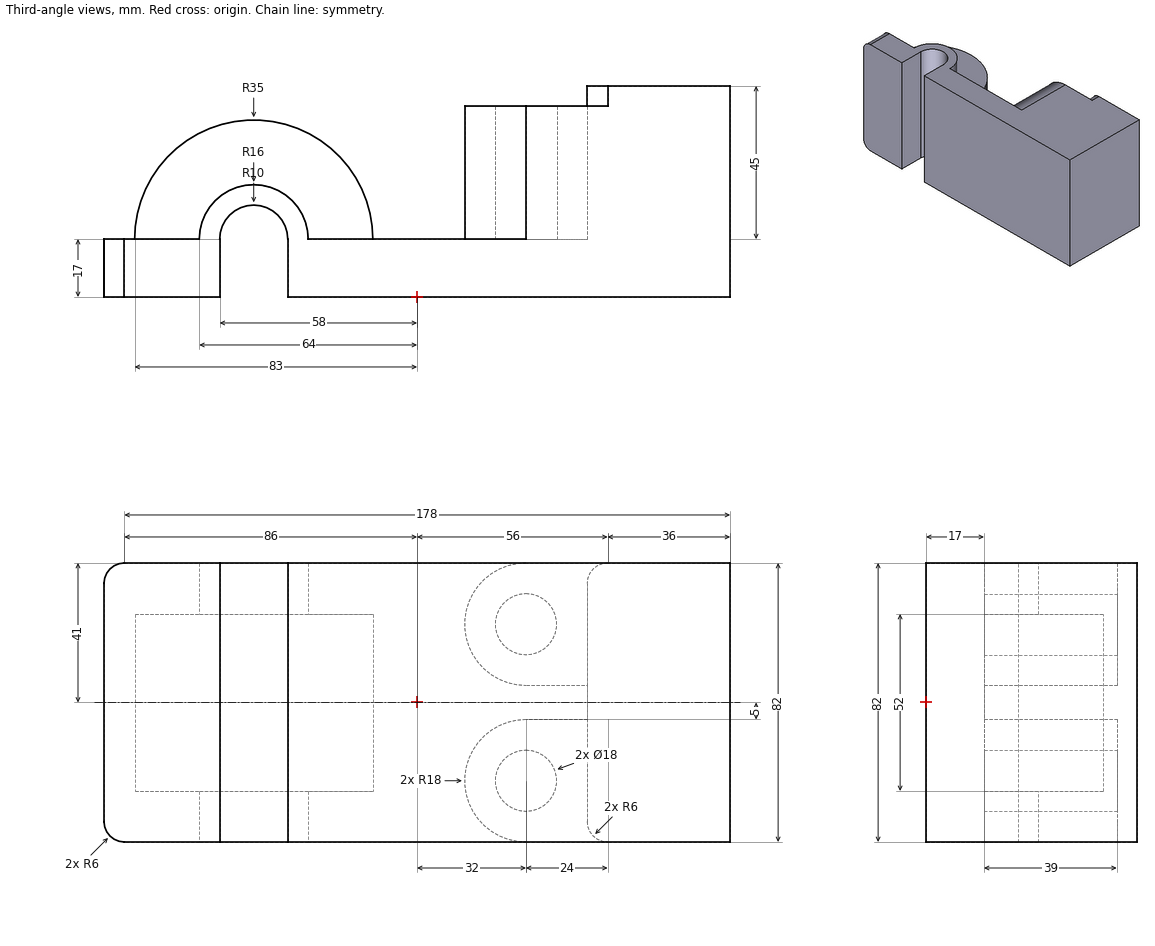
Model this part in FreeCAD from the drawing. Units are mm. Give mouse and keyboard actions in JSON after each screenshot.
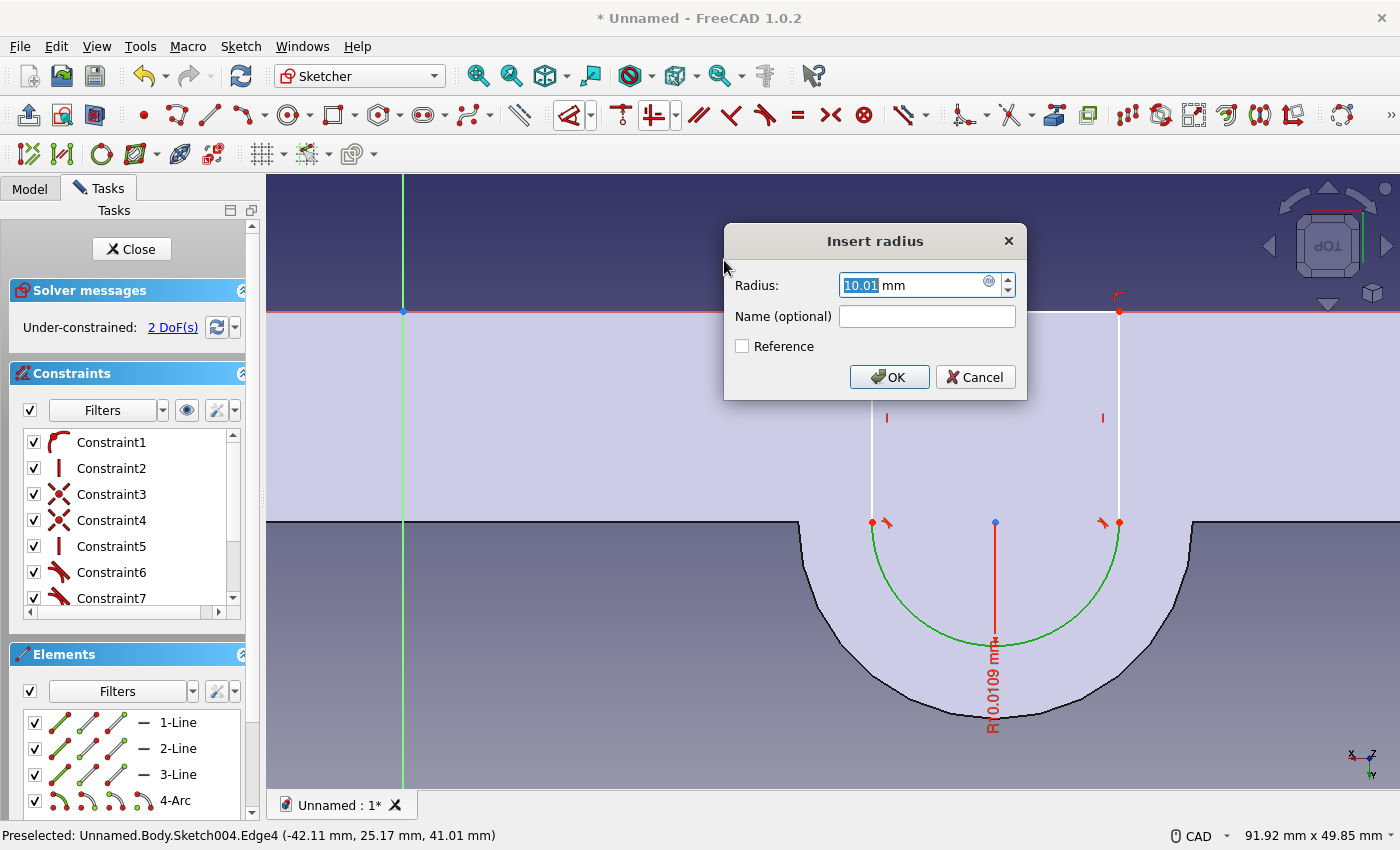
{"action": "type", "text": "10"}
{"action": "key", "text": "Return"}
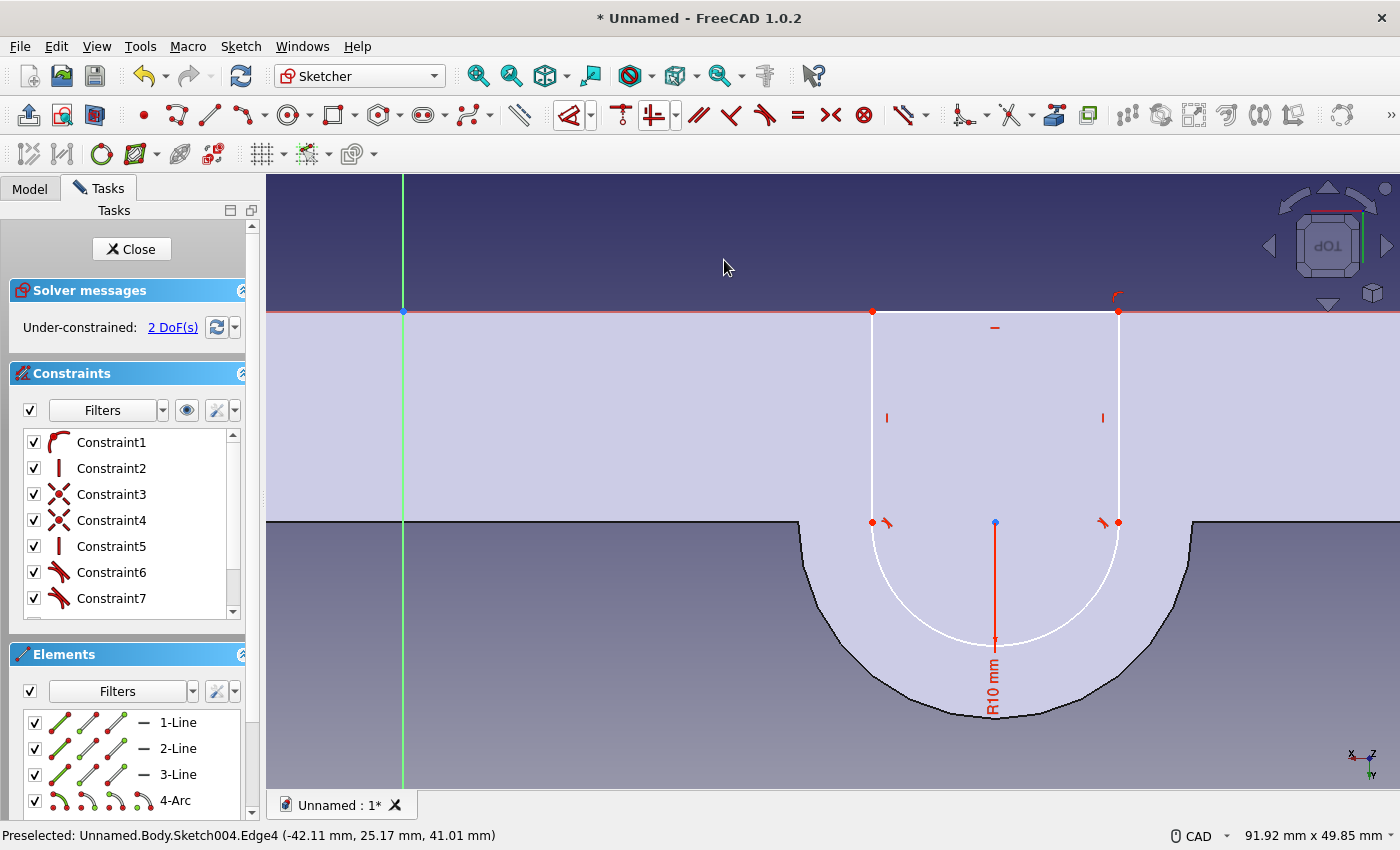
{"action": "left_click", "coordinate": [1119, 459]}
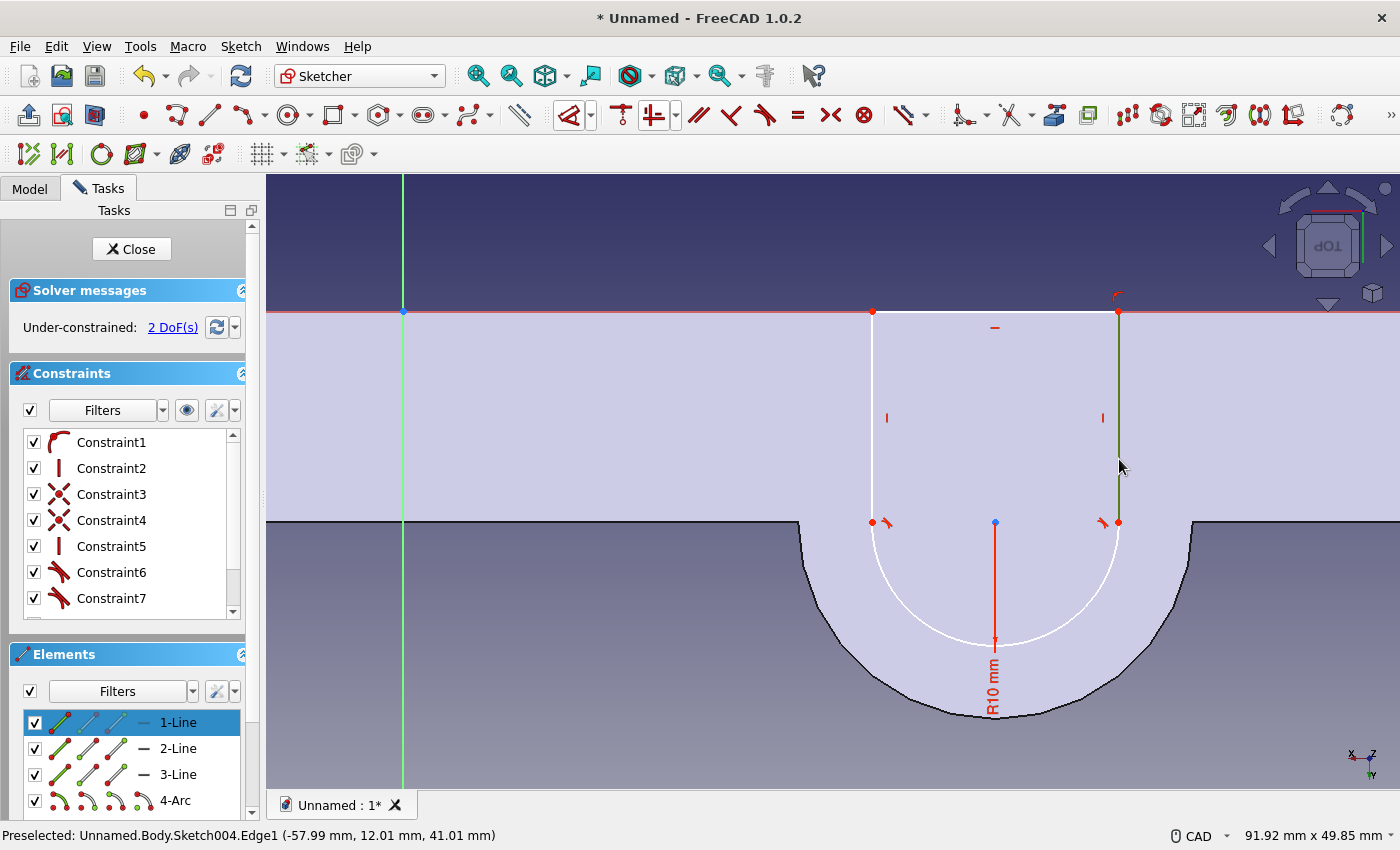
{"action": "left_click", "coordinate": [590, 116]}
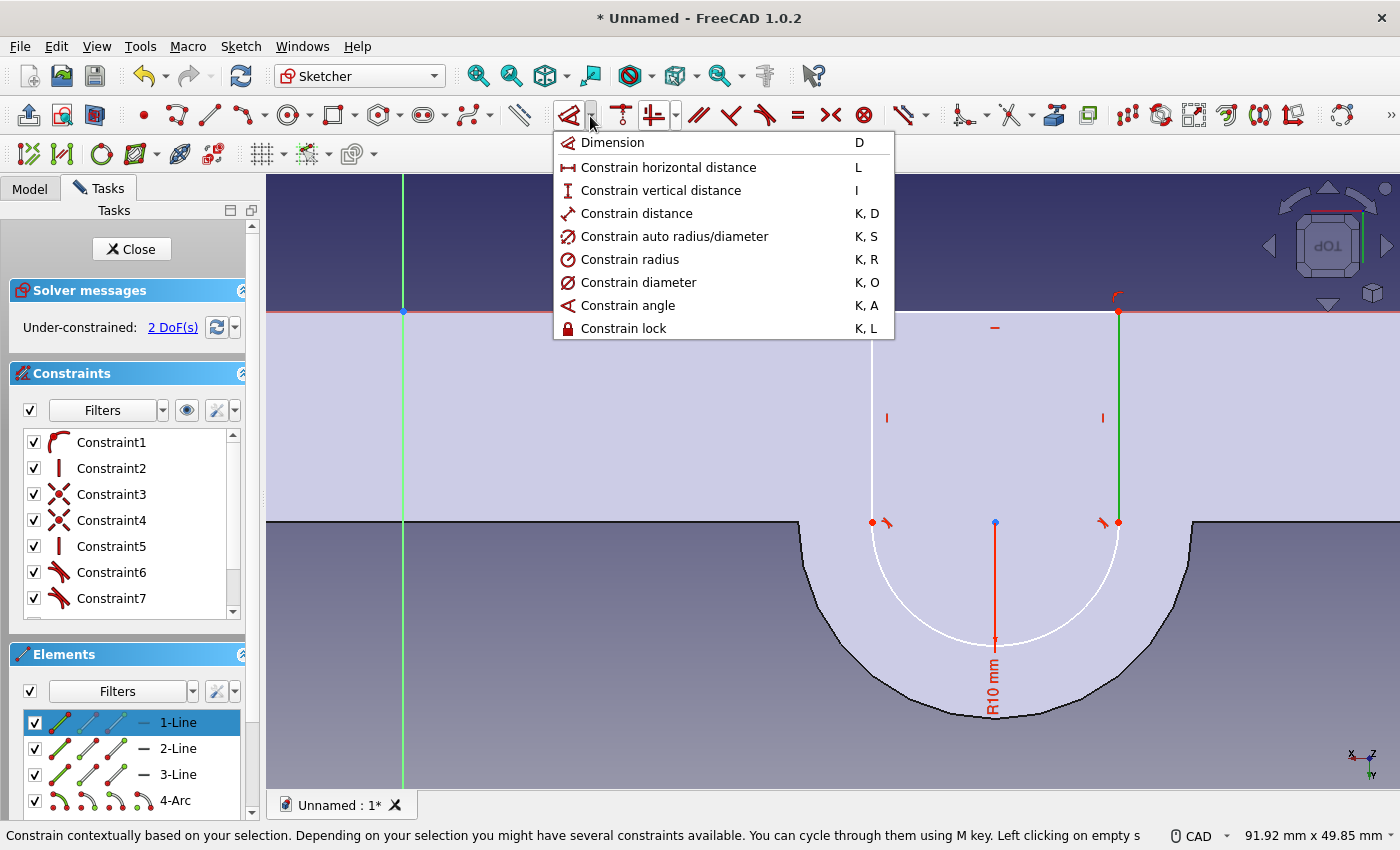
{"action": "left_click", "coordinate": [724, 190]}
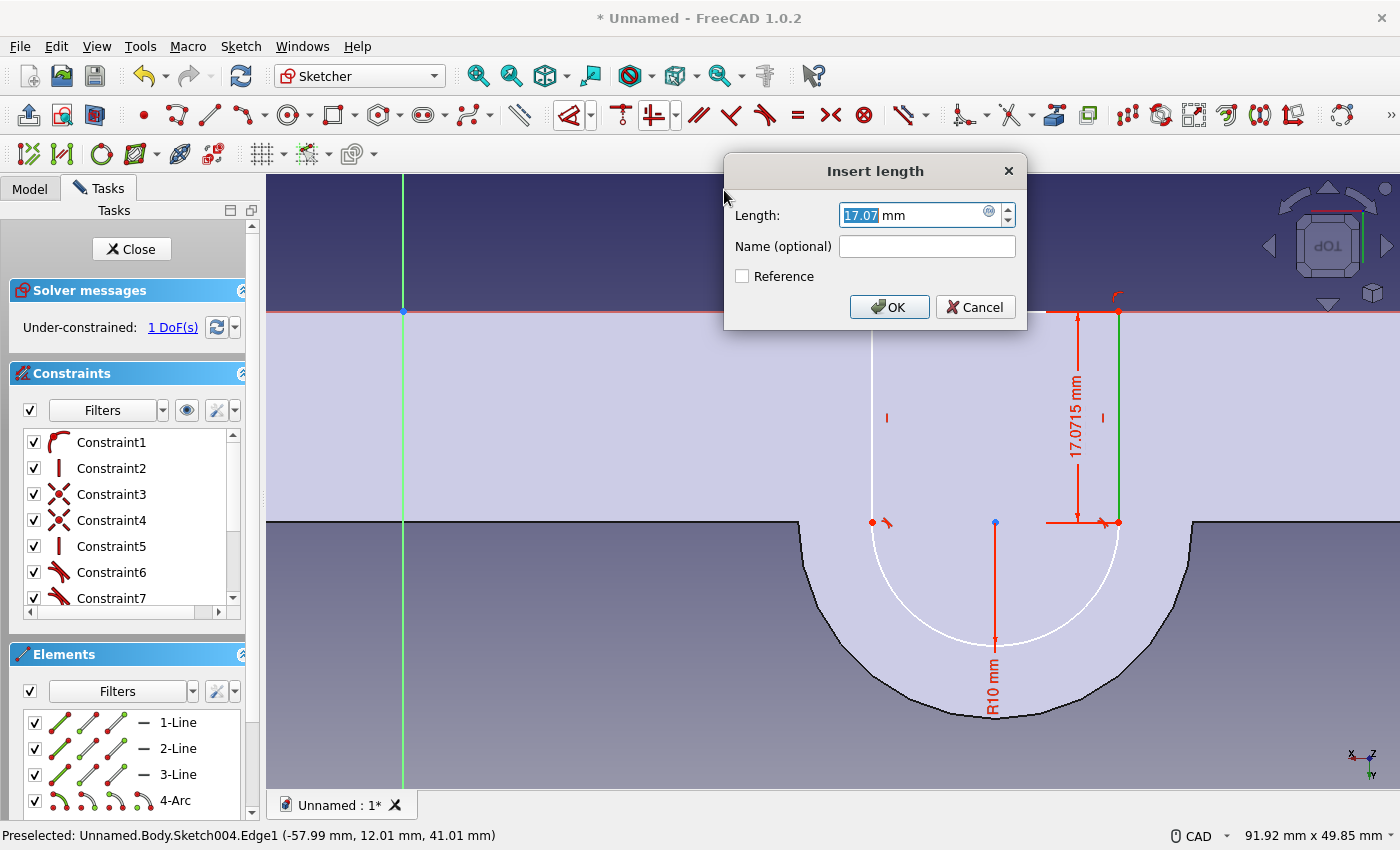
{"action": "type", "text": "17"}
{"action": "key", "text": "Return"}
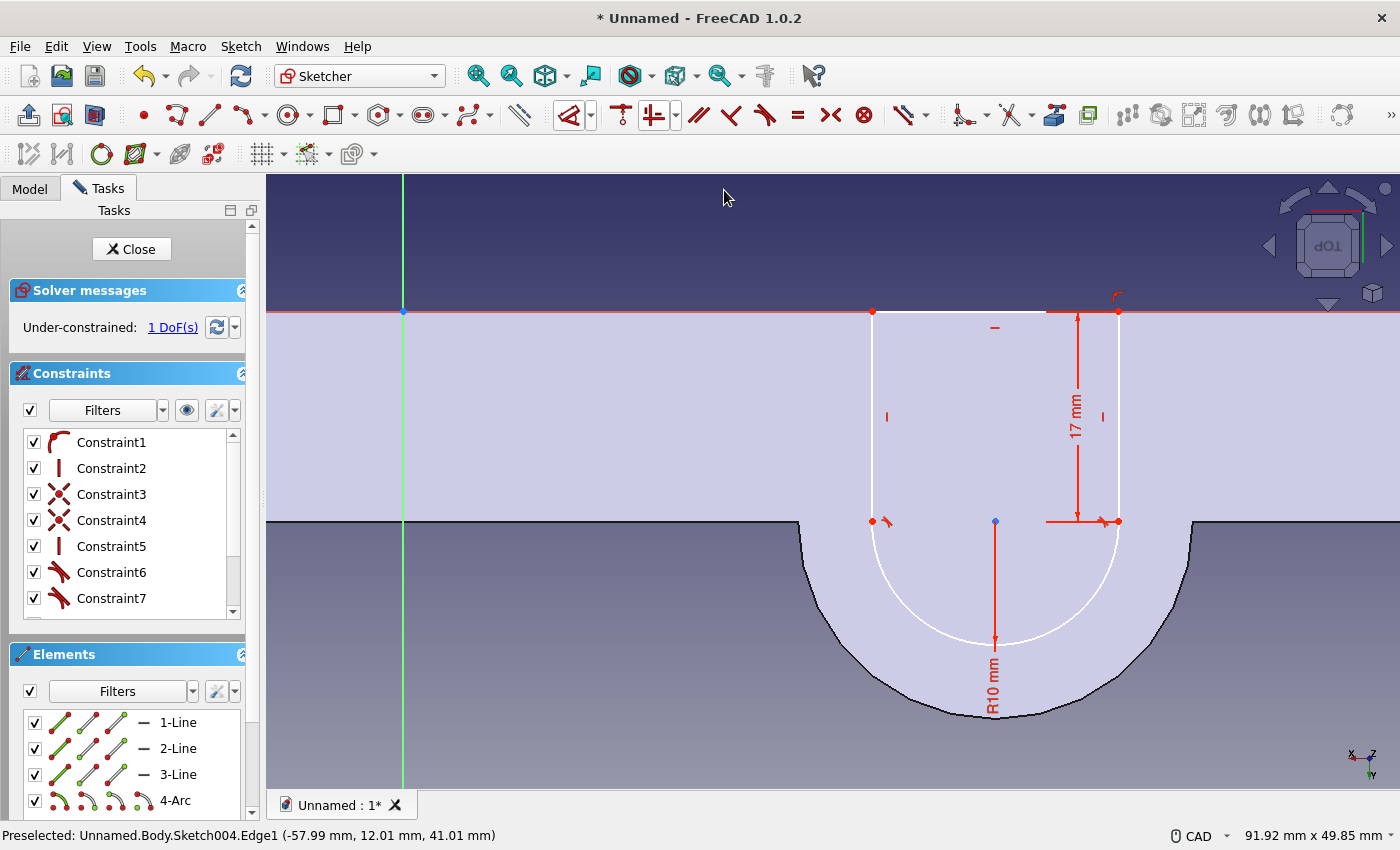
{"action": "left_click", "coordinate": [1119, 522]}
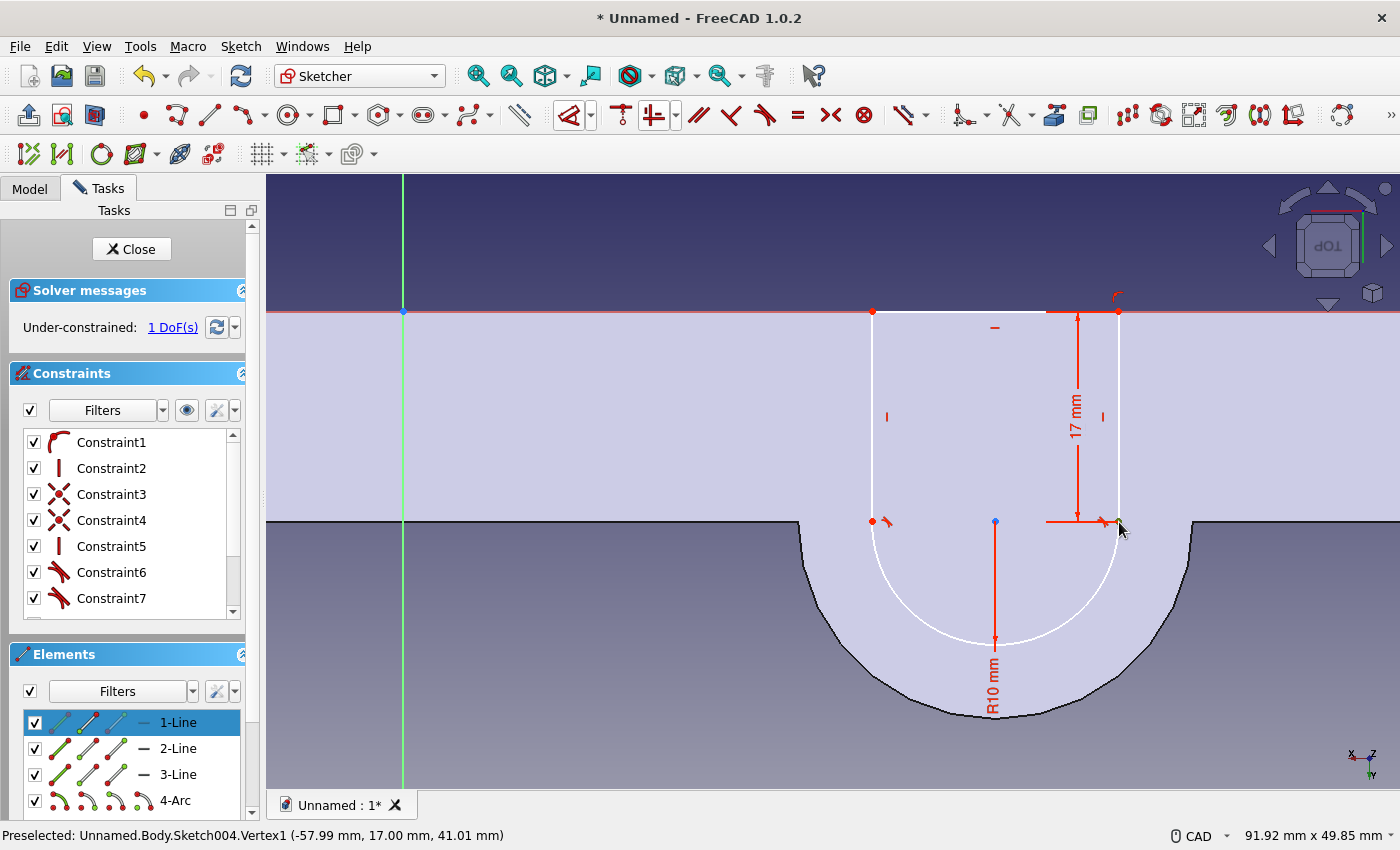
{"action": "left_click", "coordinate": [590, 116]}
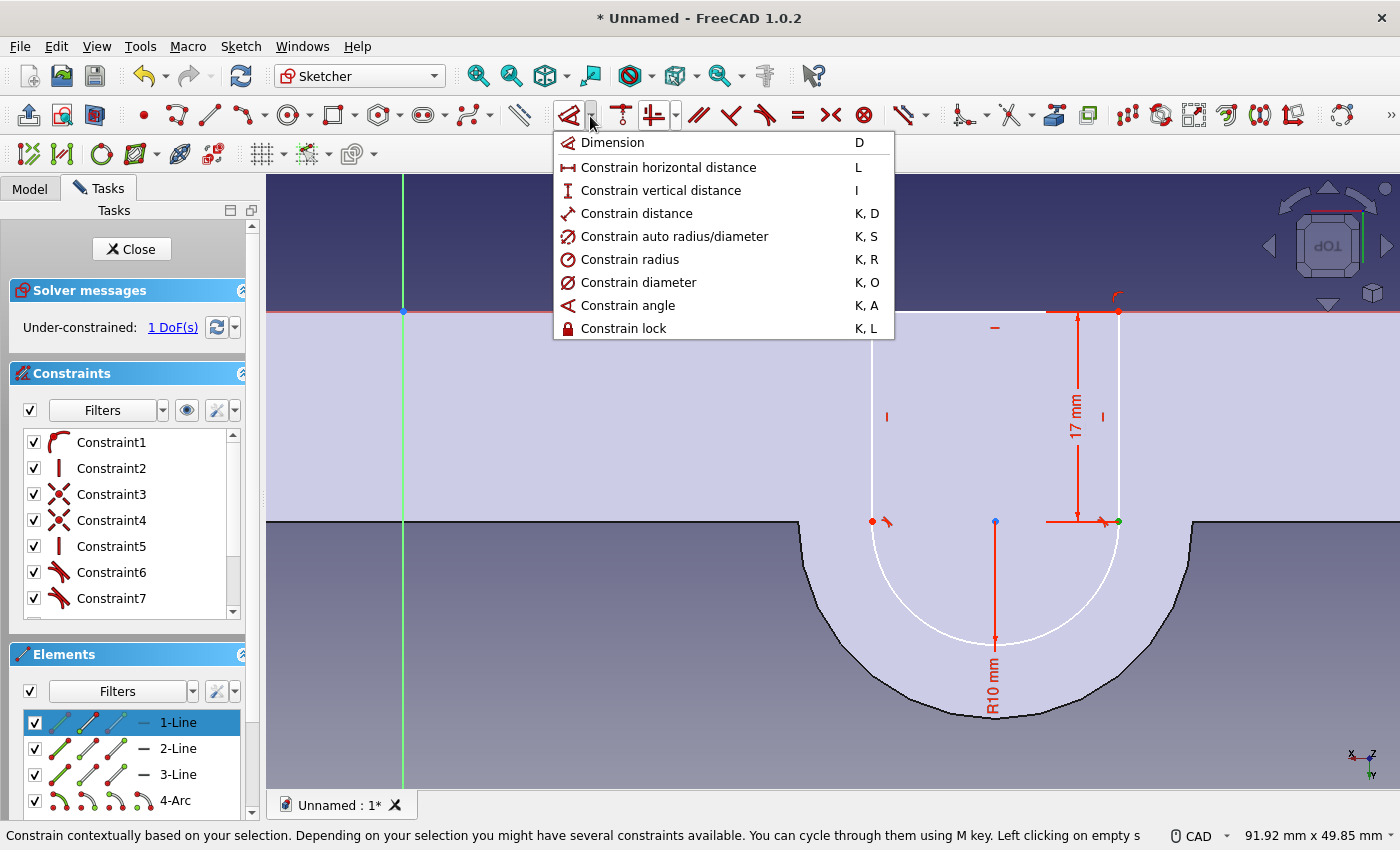
{"action": "left_click", "coordinate": [724, 168]}